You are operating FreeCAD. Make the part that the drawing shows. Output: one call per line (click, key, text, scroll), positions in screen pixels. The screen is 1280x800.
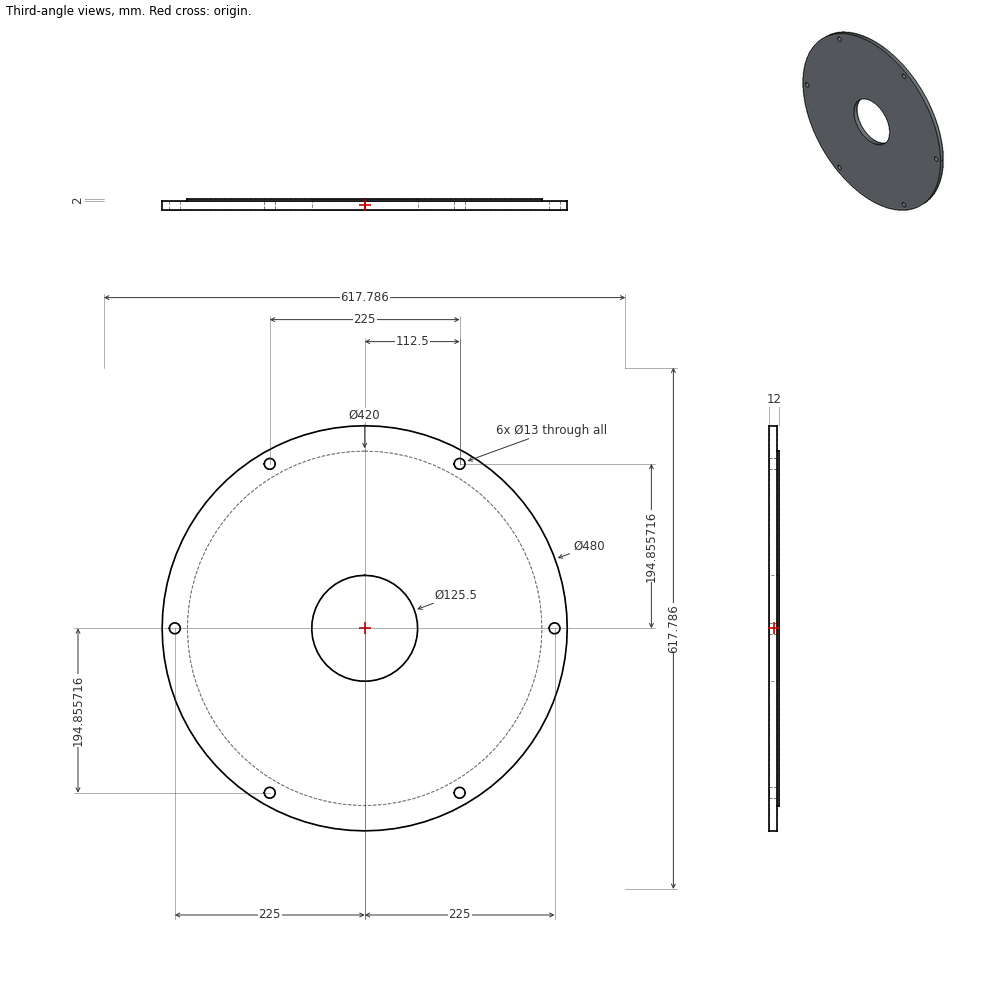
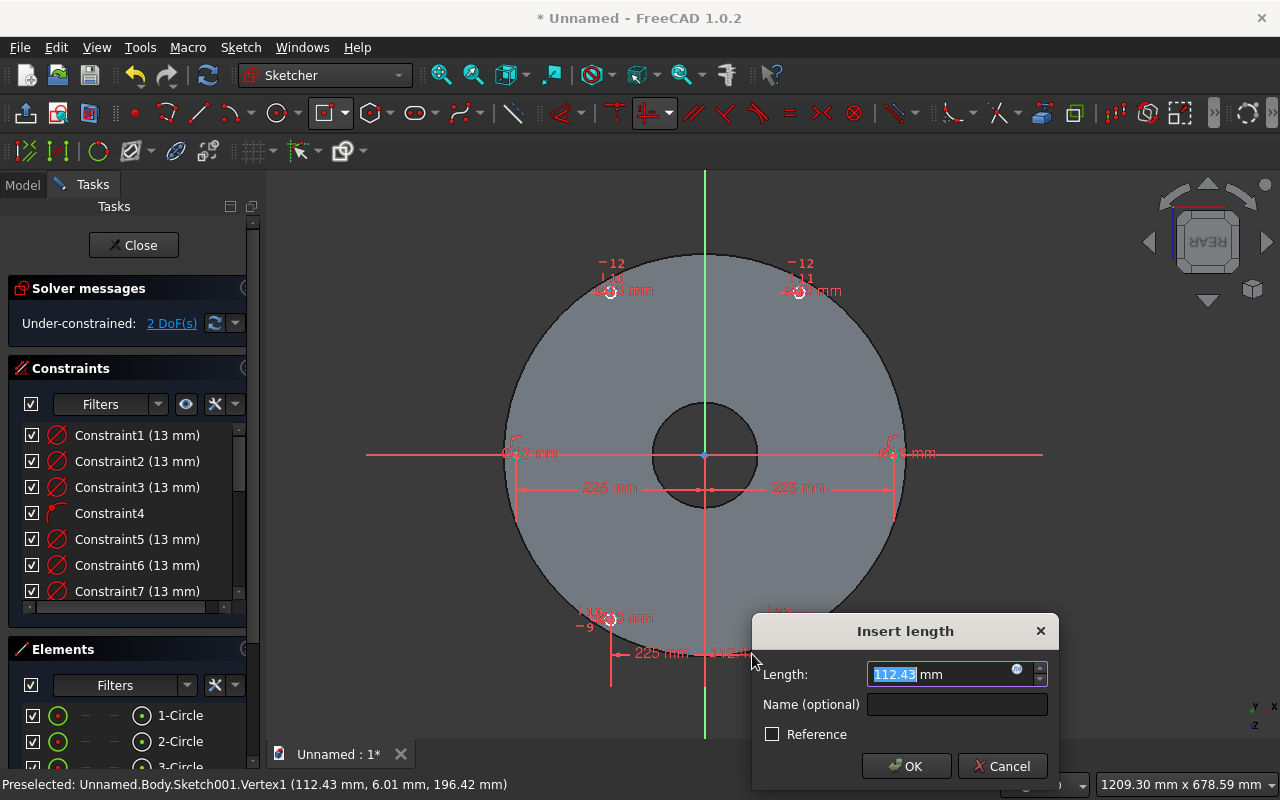
text(112.5)
key(Return)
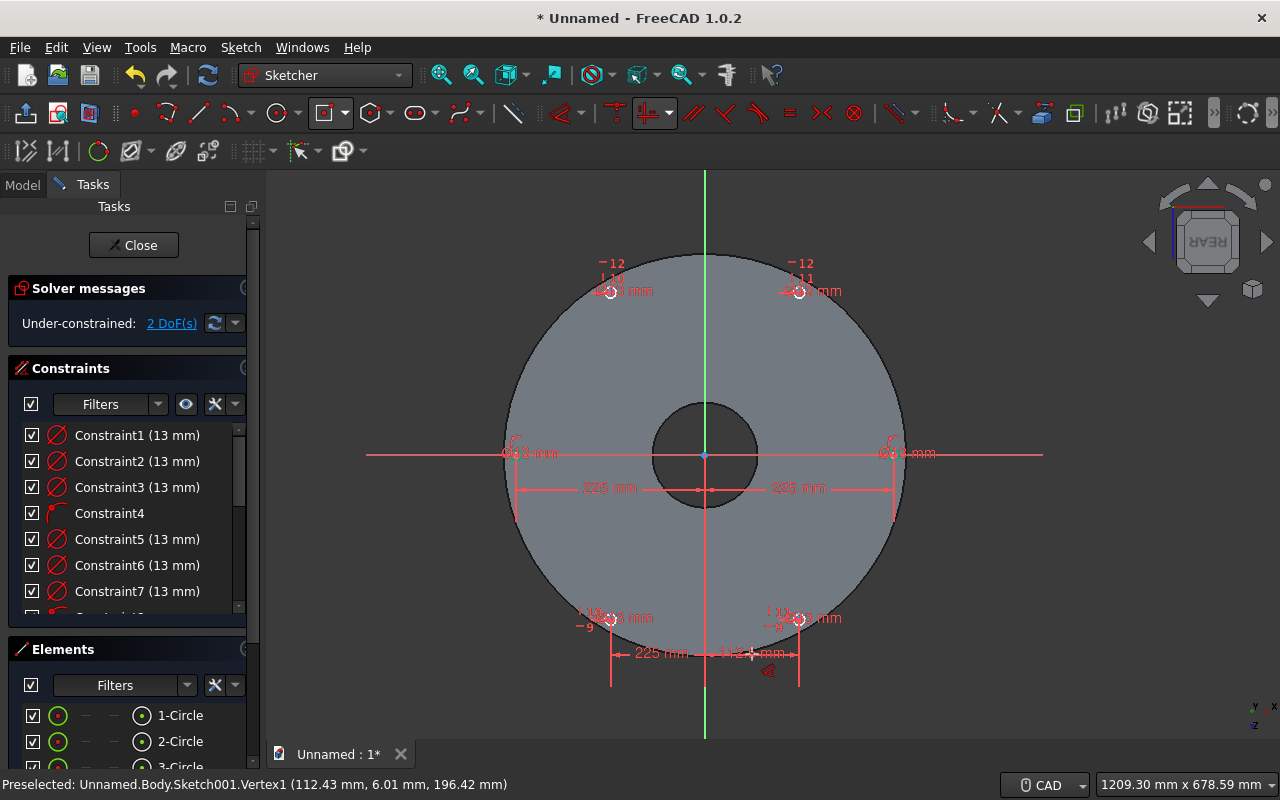
click(799, 620)
click(833, 538)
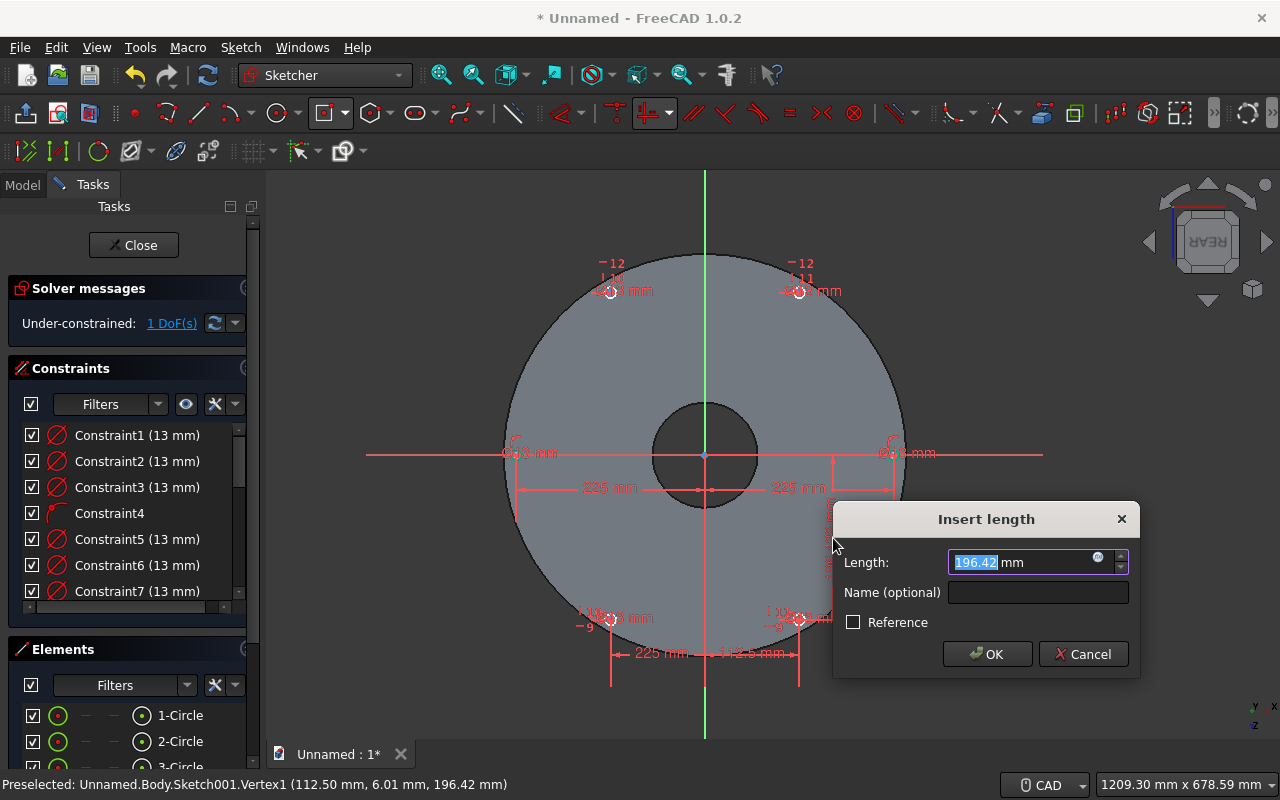
text(194.855716)
key(Return)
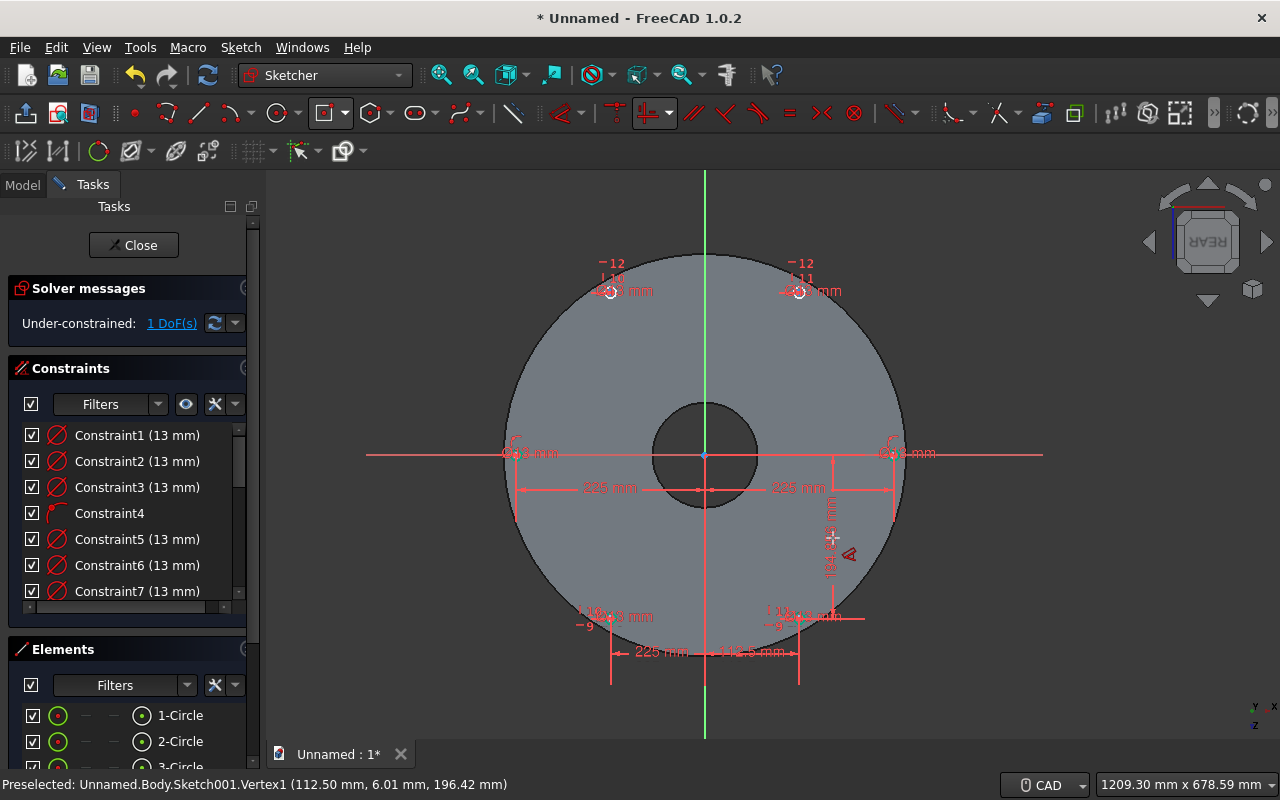
click(611, 293)
click(577, 374)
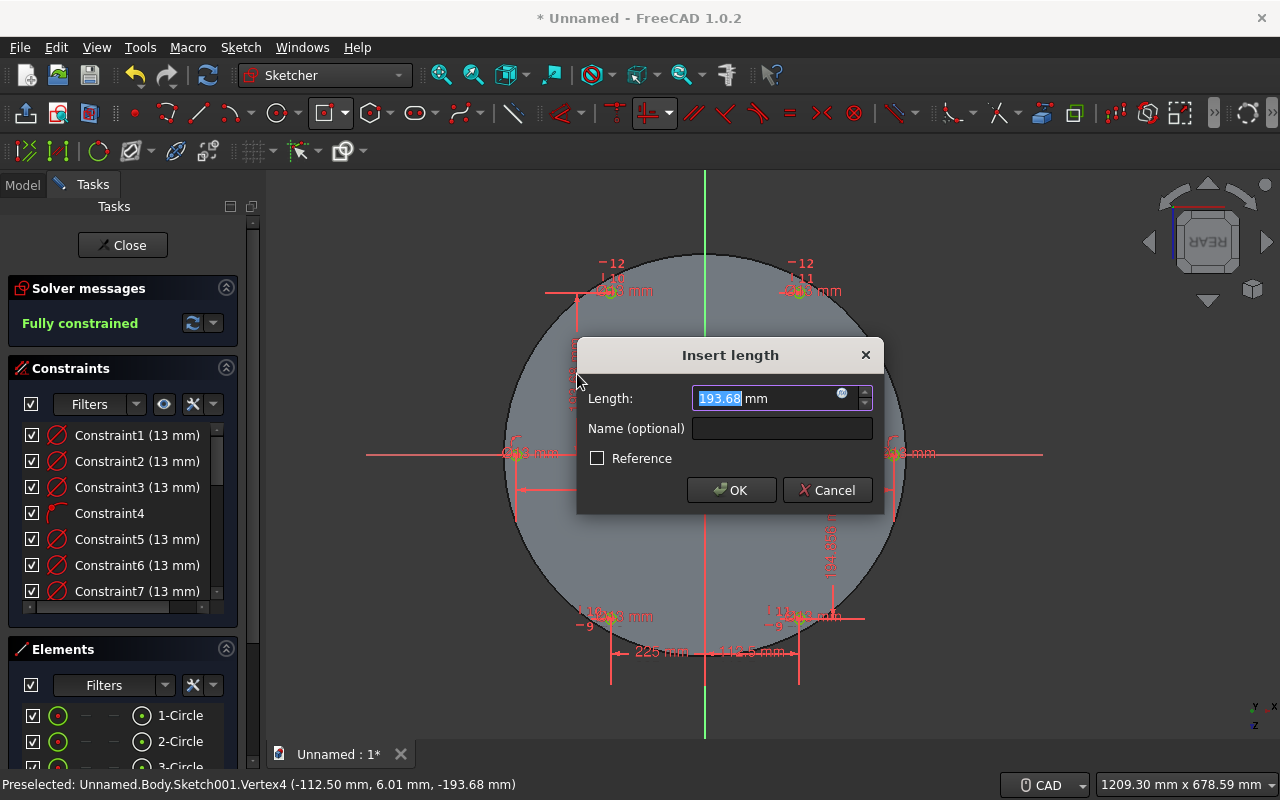
text(194.855716)
key(Return)
key(Escape)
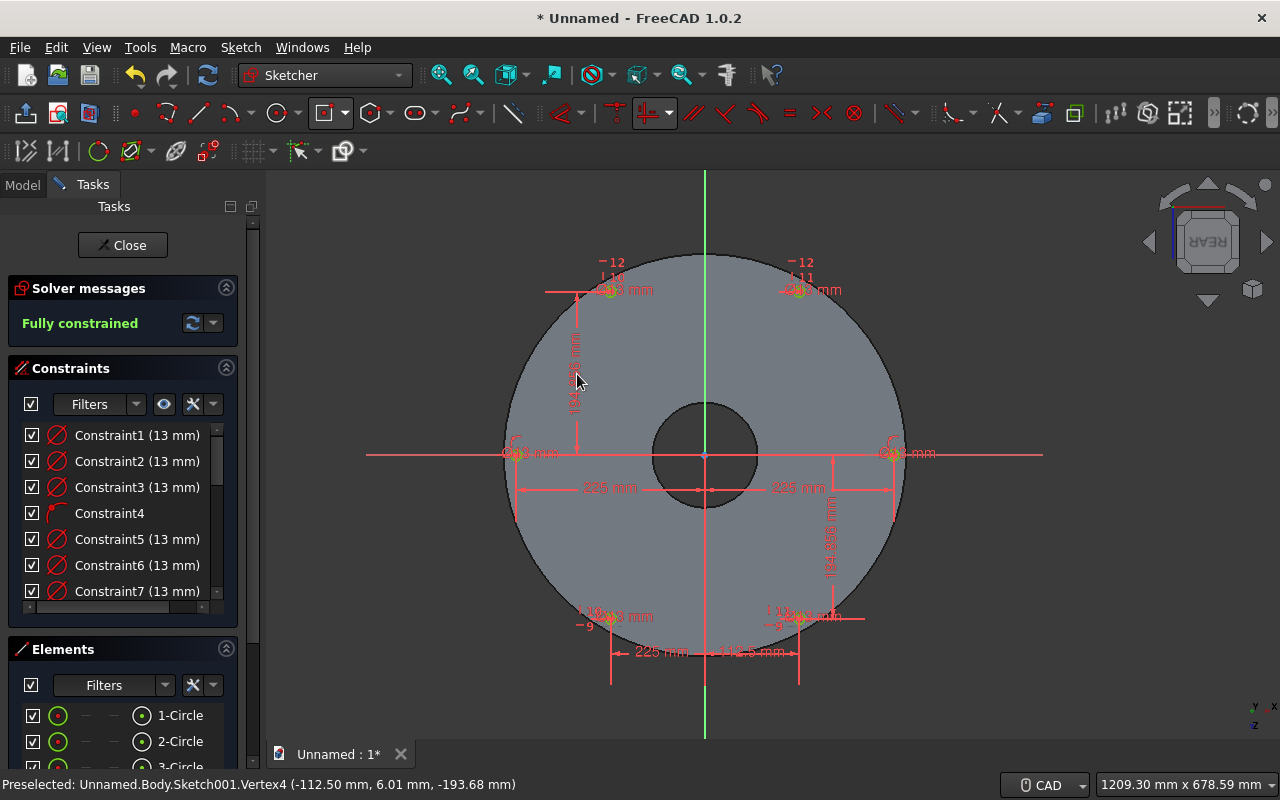
click(123, 245)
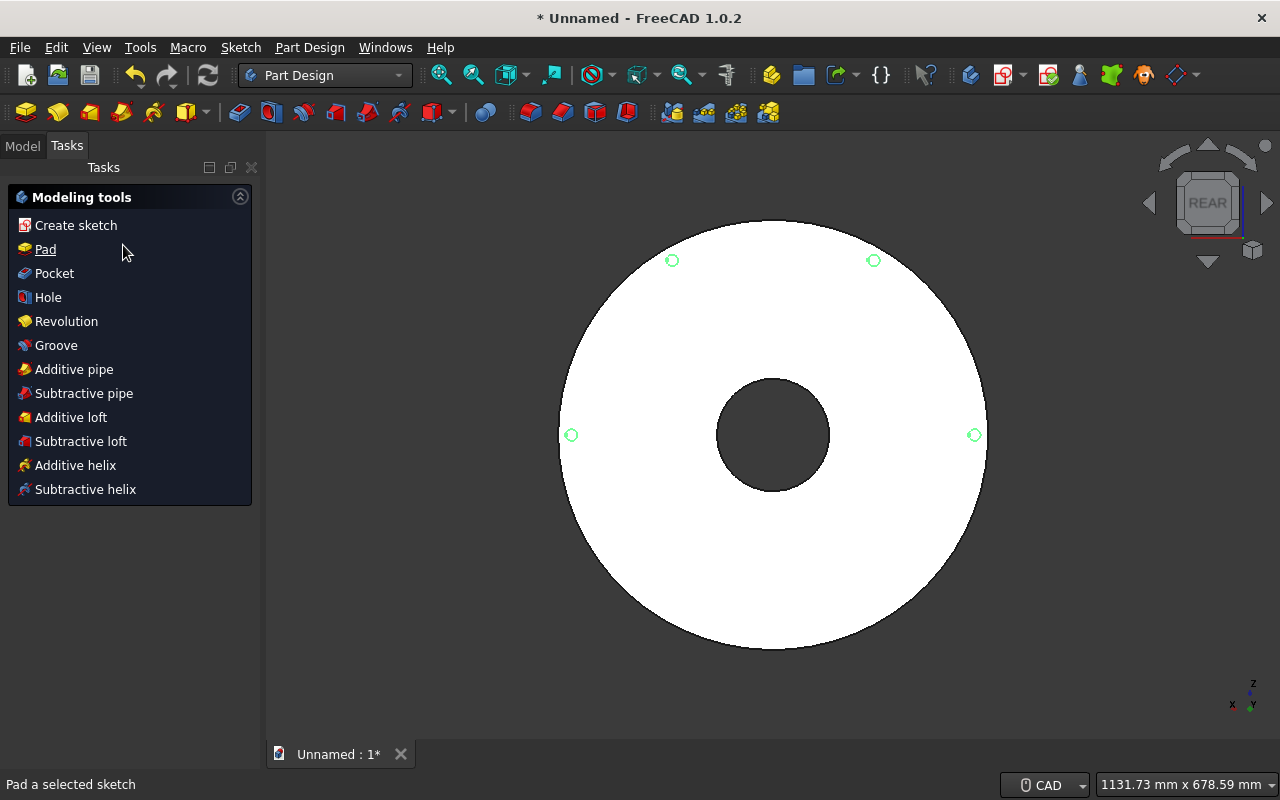
click(272, 112)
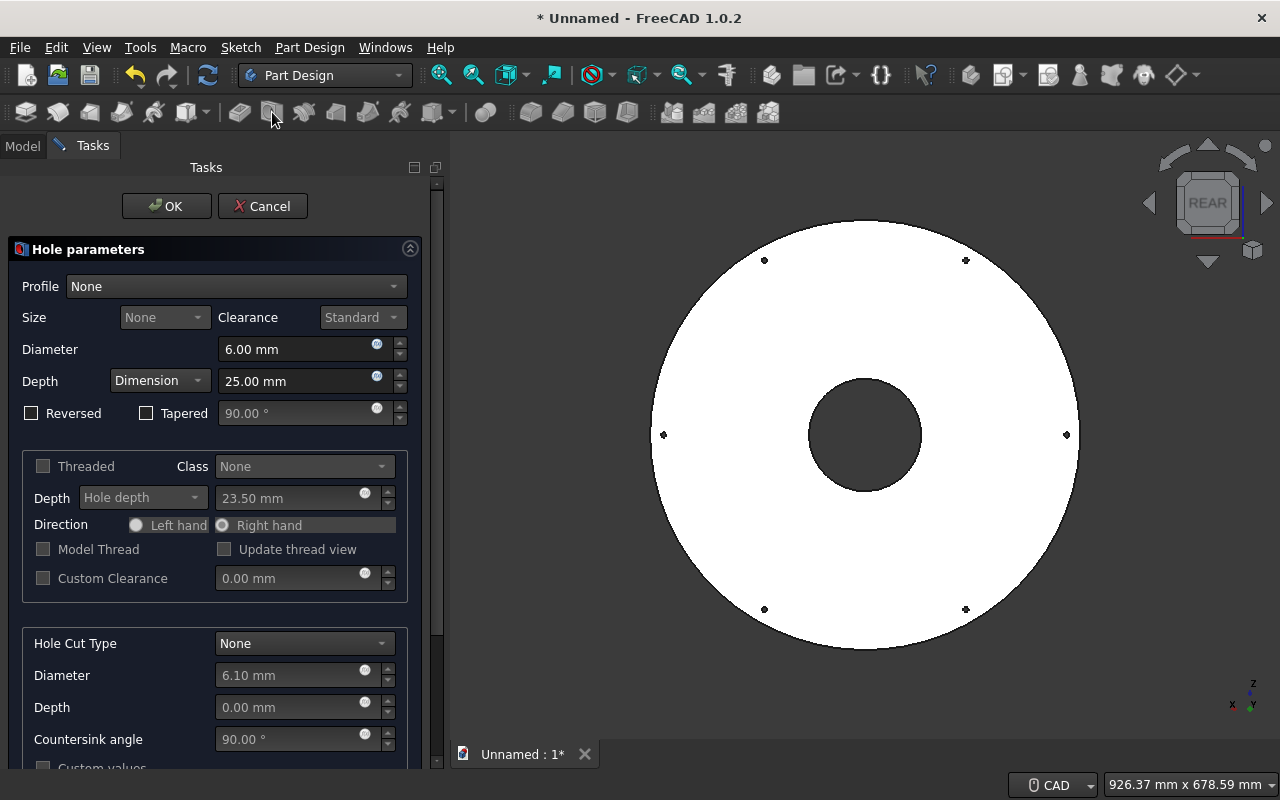
triple_click(305, 349)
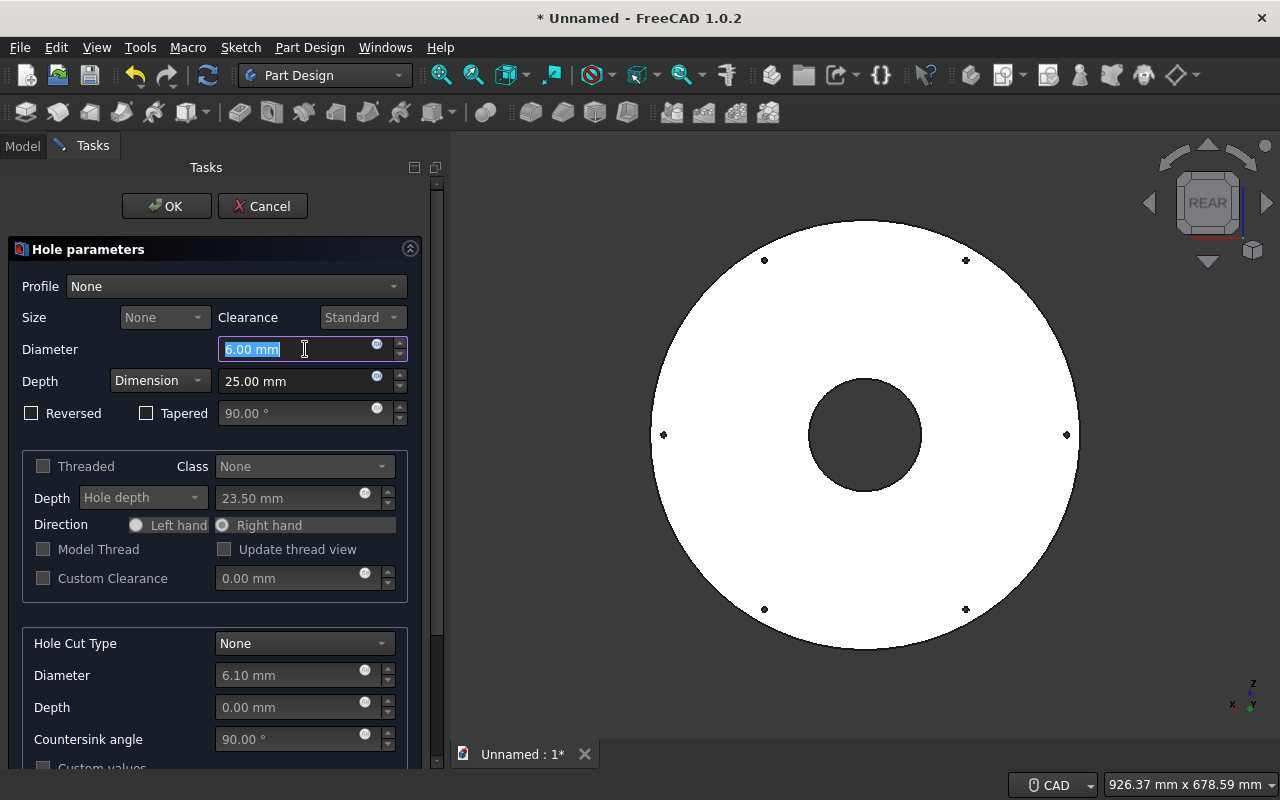
text(13)
key(Tab)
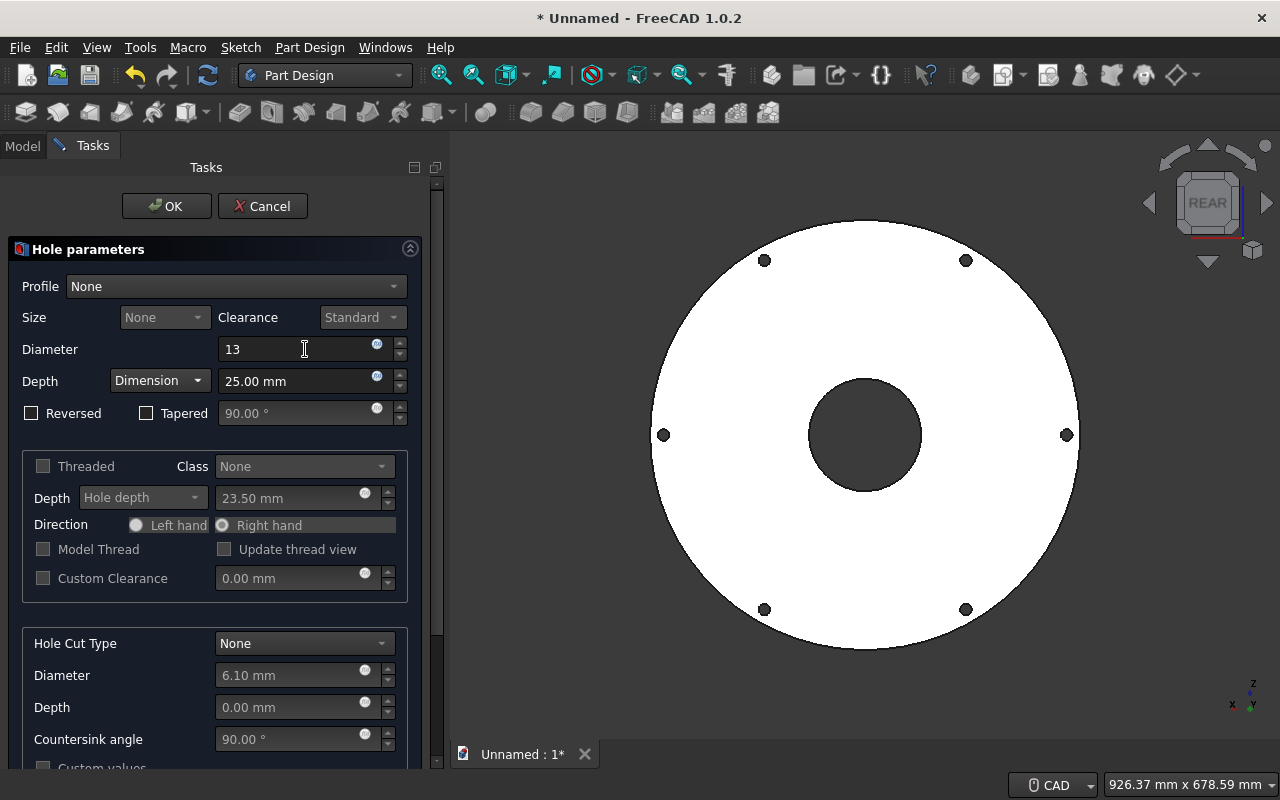
click(161, 380)